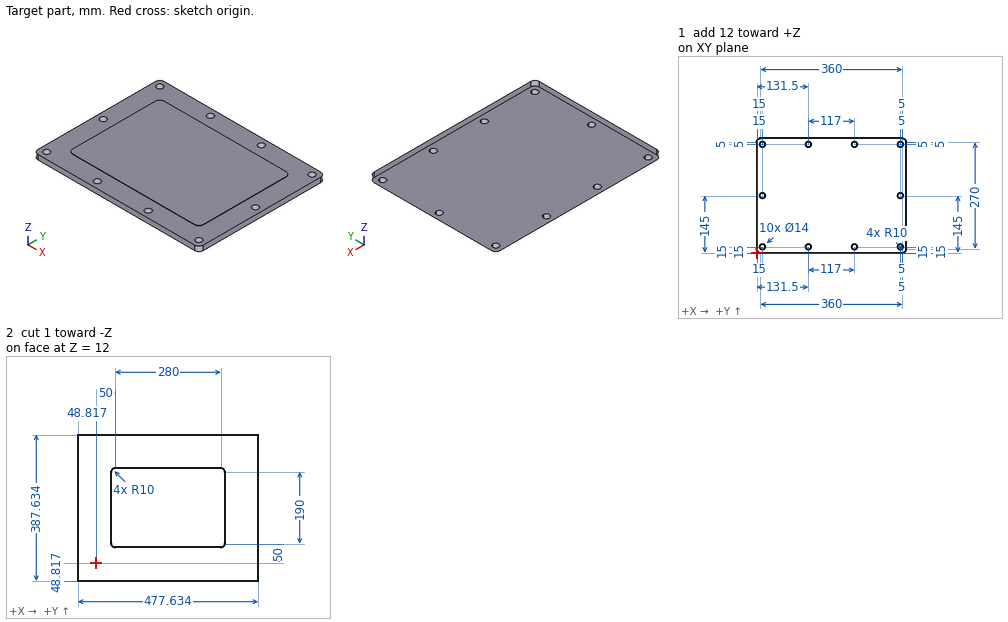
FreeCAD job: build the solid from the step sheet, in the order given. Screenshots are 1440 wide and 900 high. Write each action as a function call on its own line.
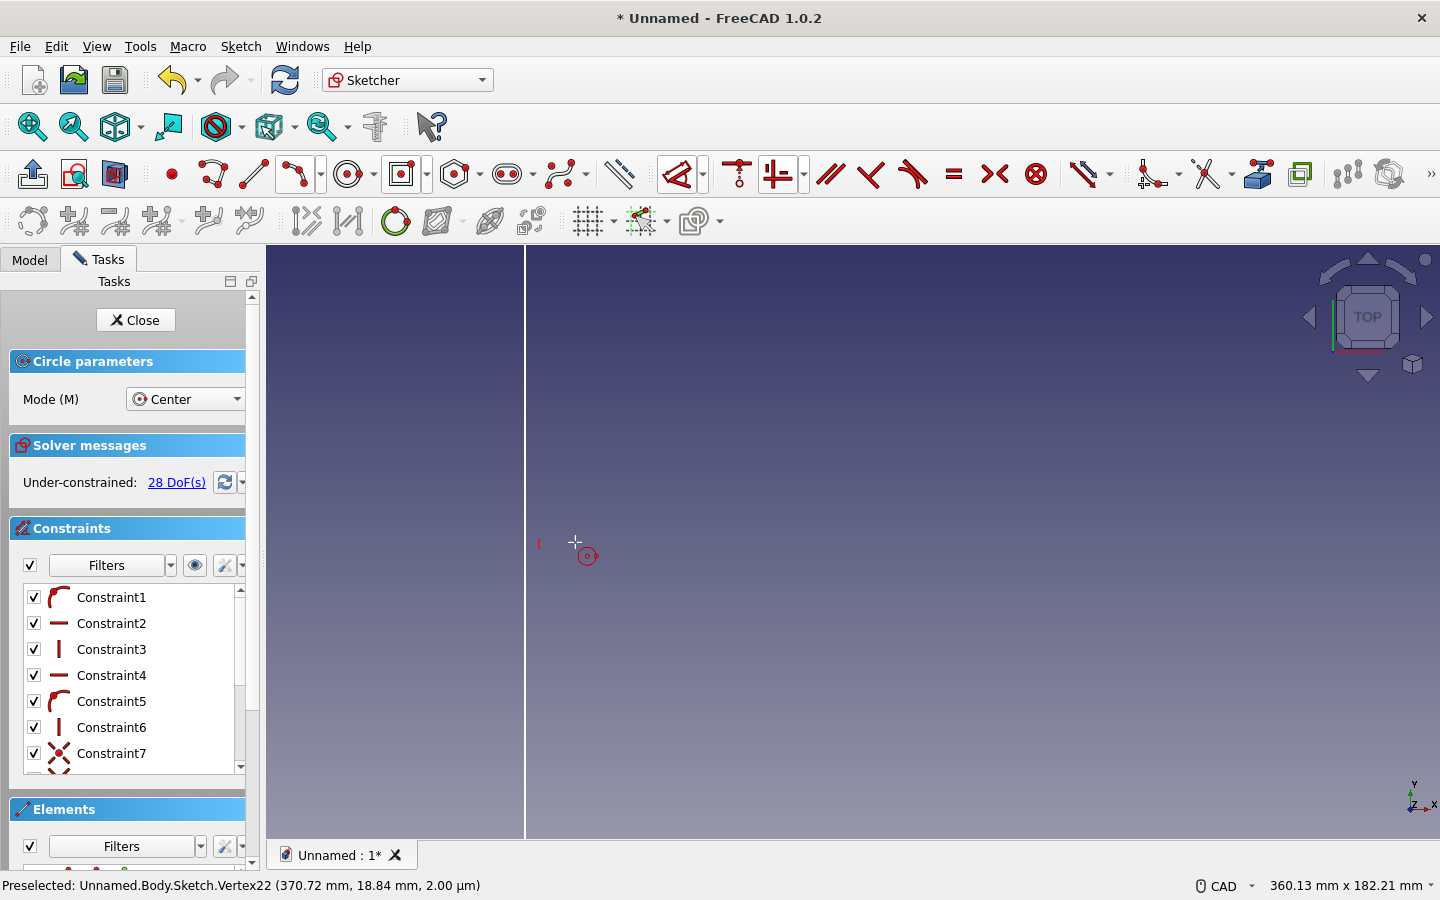
click(574, 542)
click(590, 526)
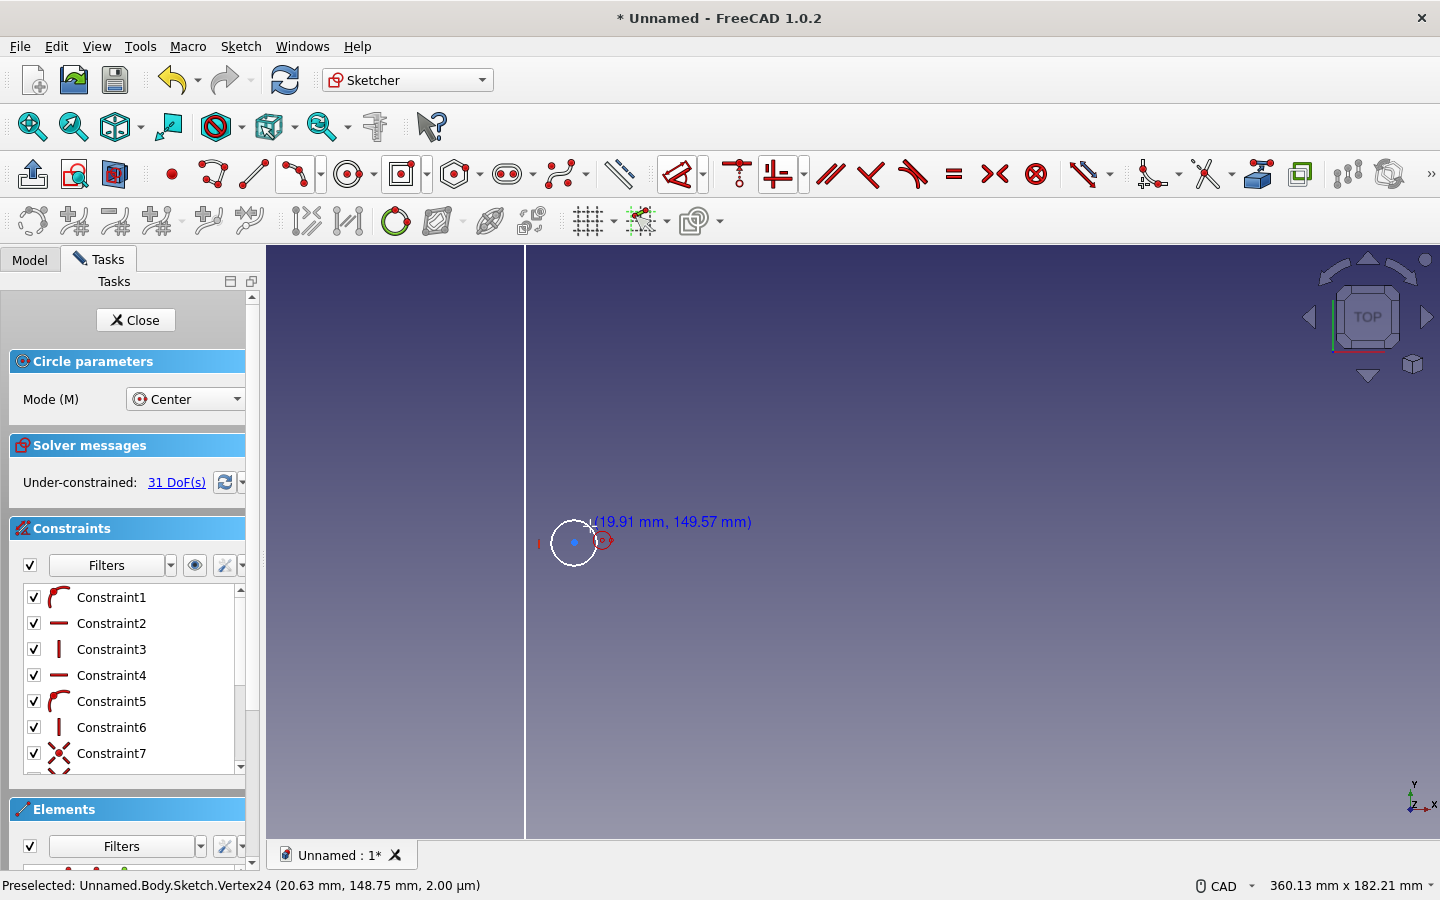
scroll(575, 542, down, 5)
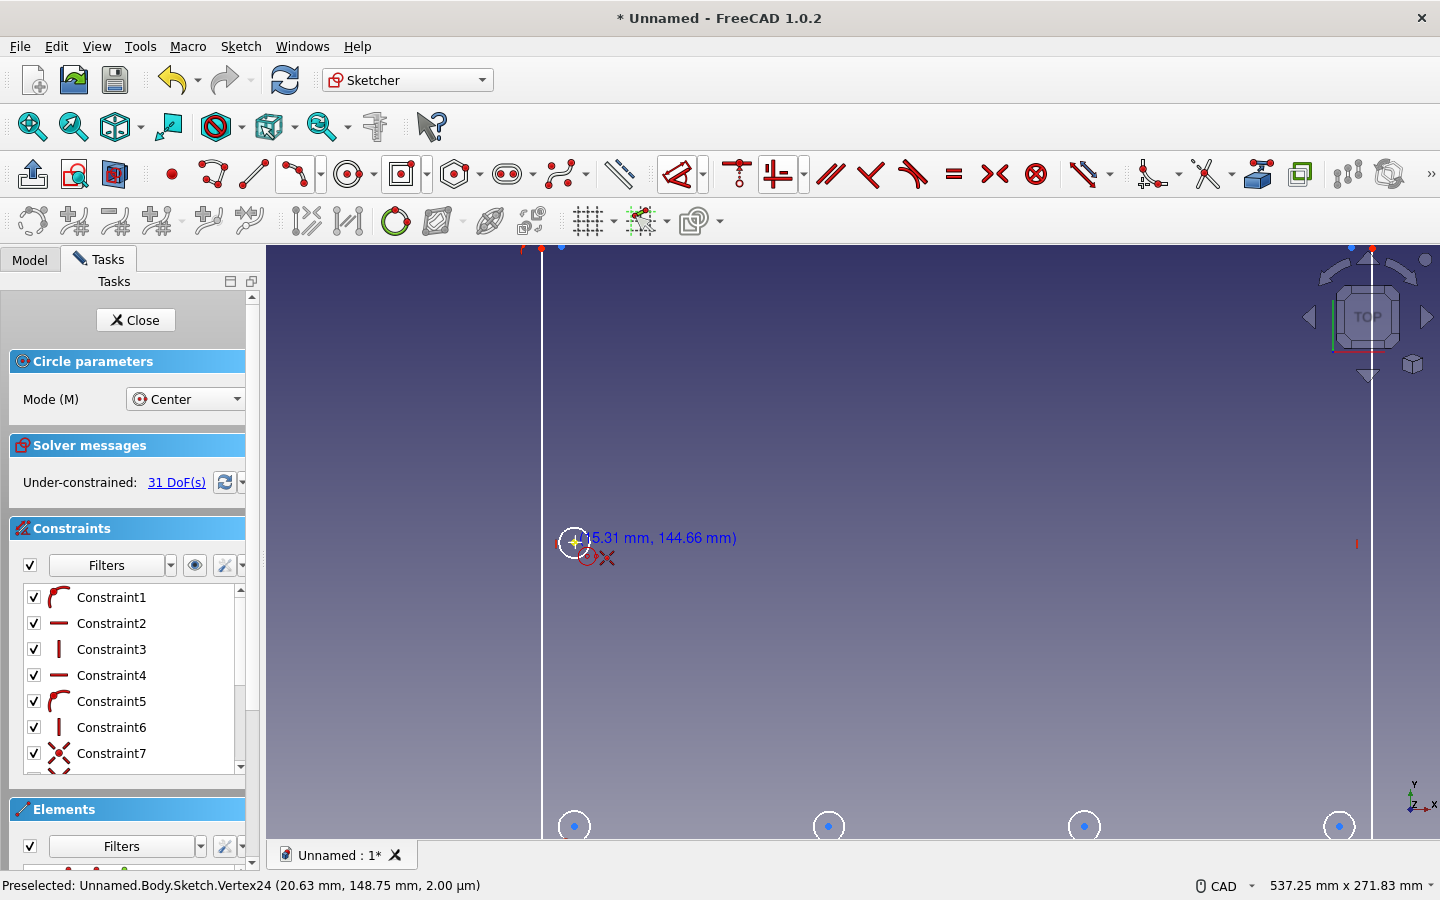
scroll(575, 386, up, 5)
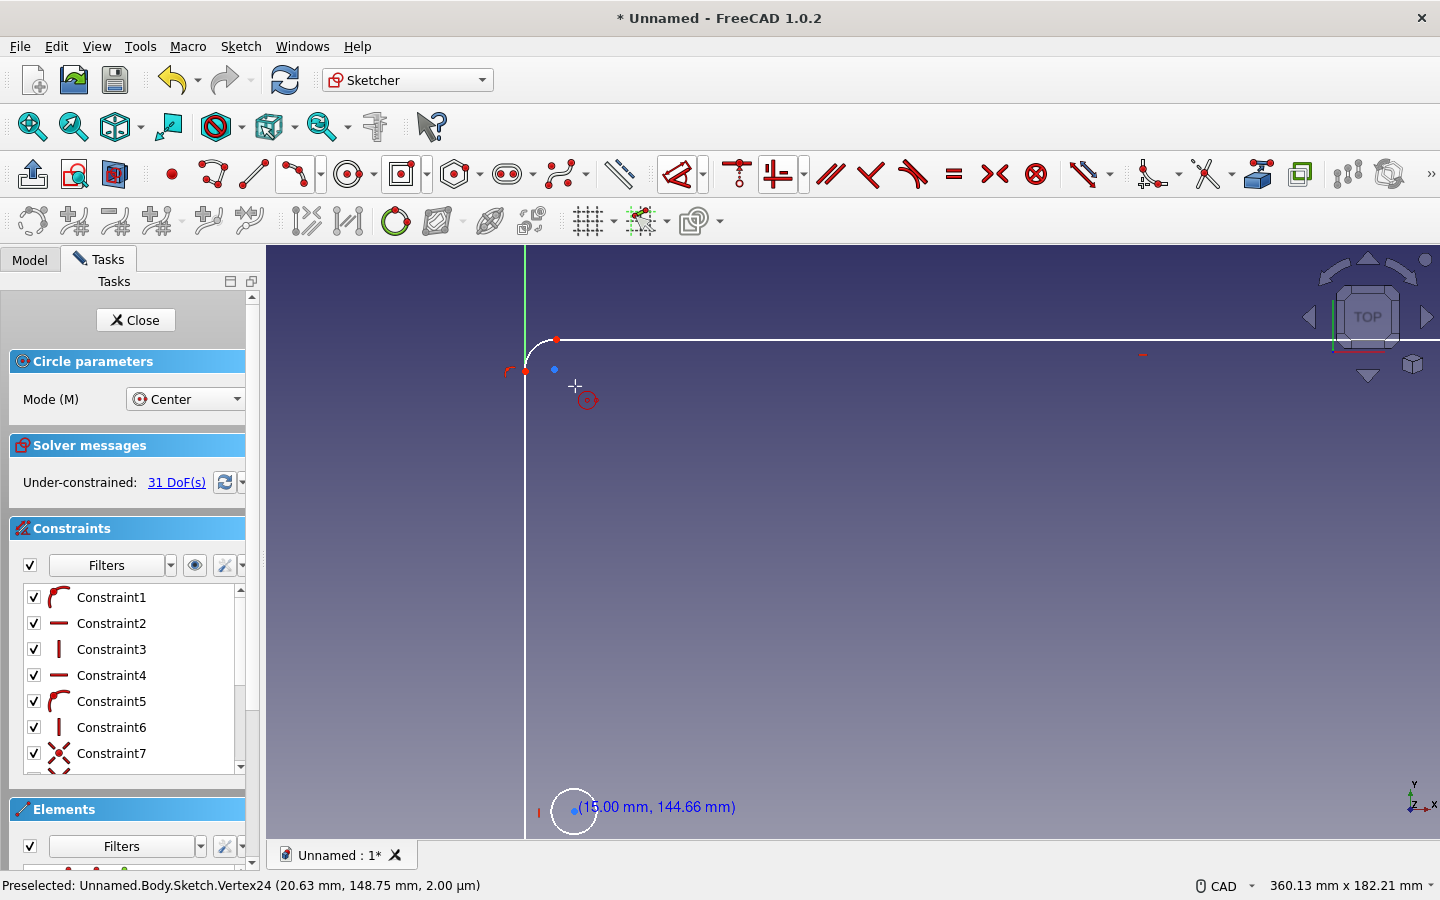
click(574, 387)
click(590, 370)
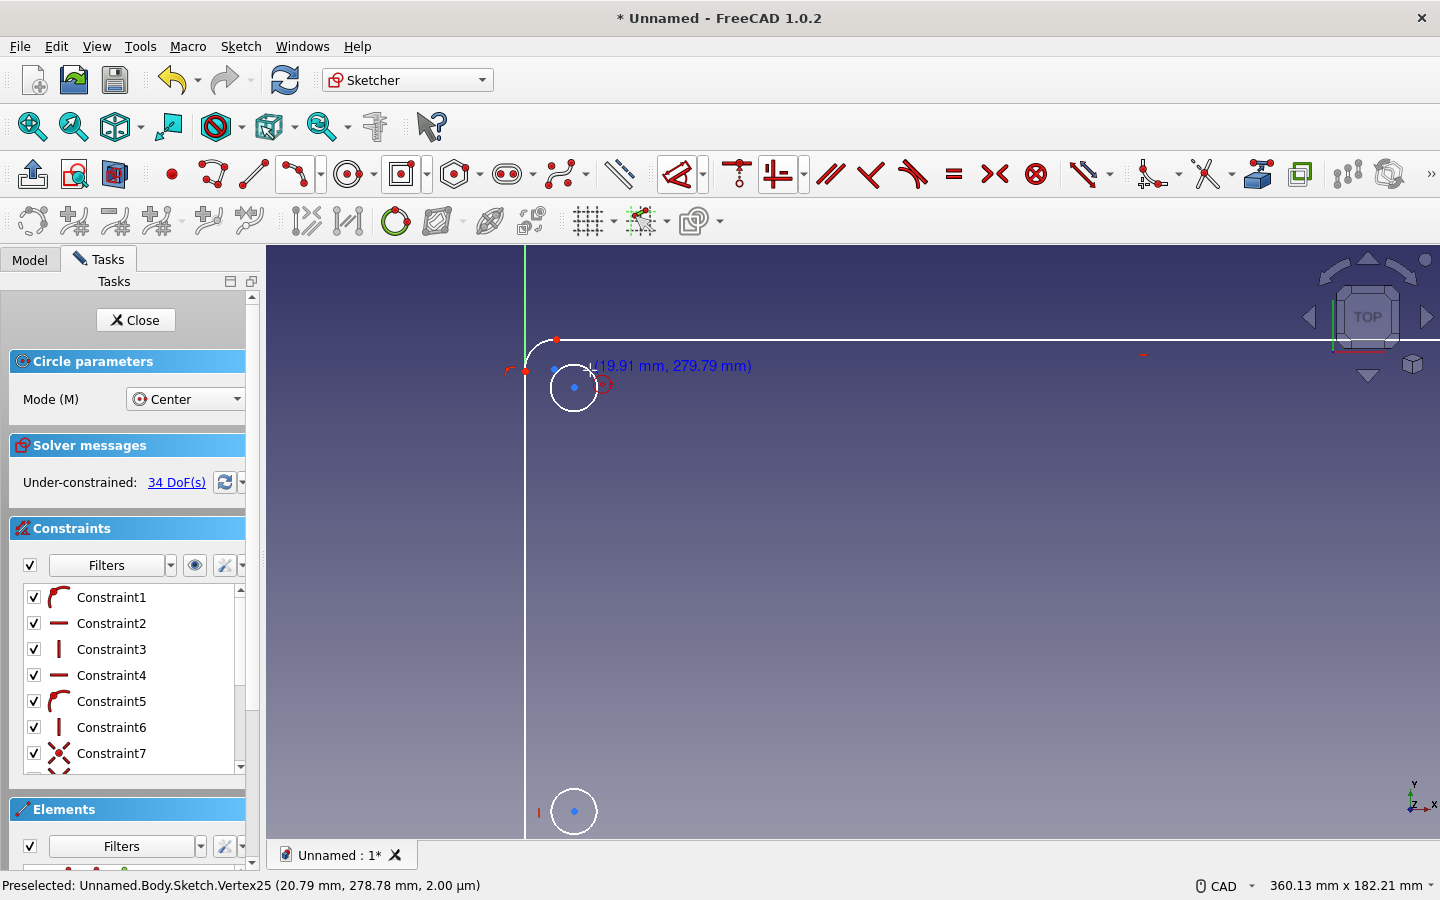
click(954, 387)
click(970, 370)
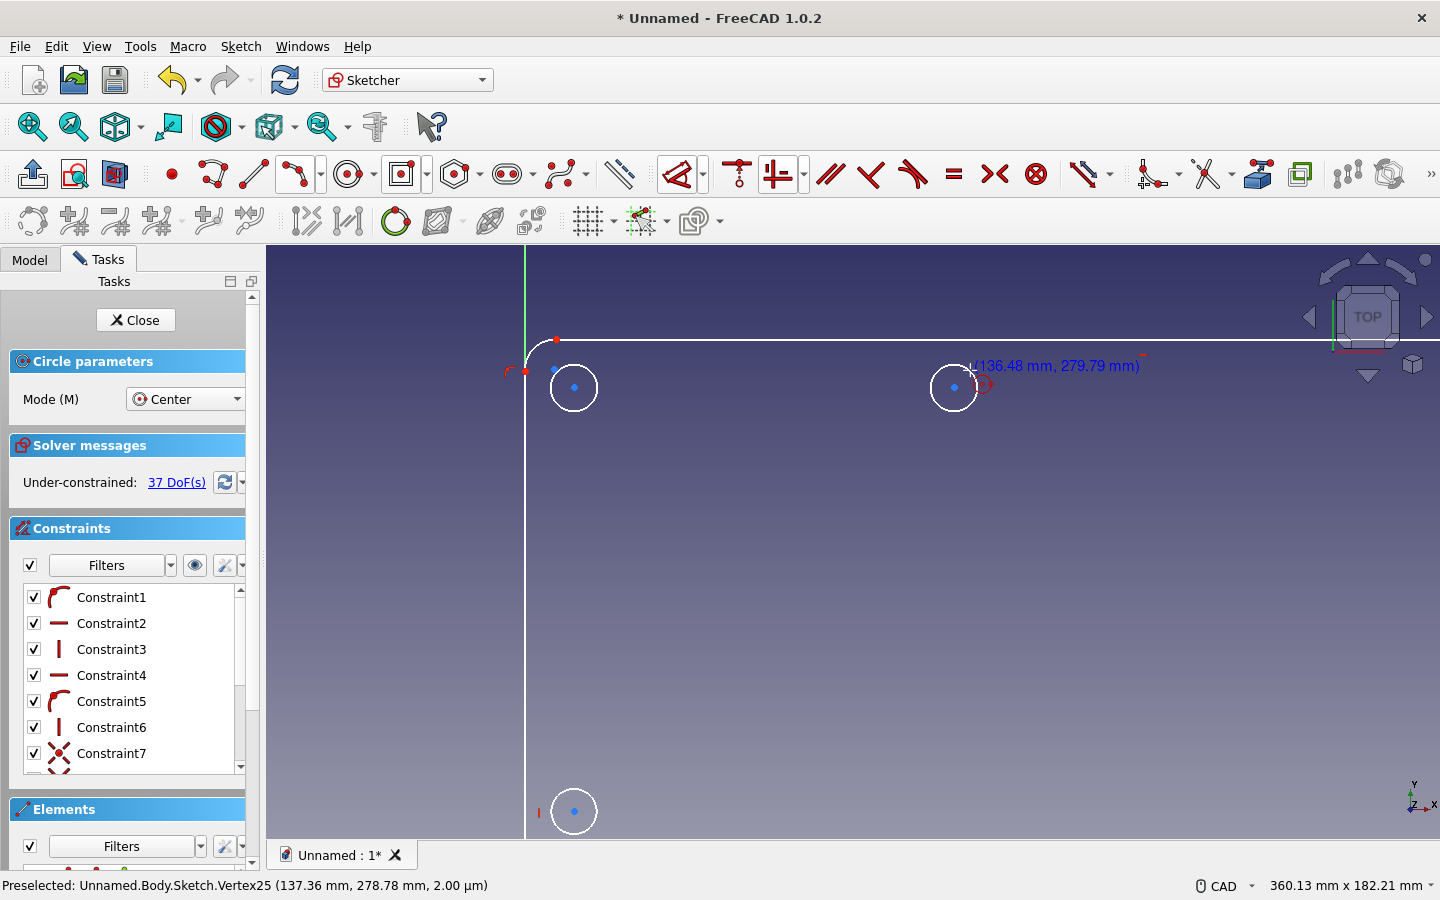
scroll(575, 386, down, 5)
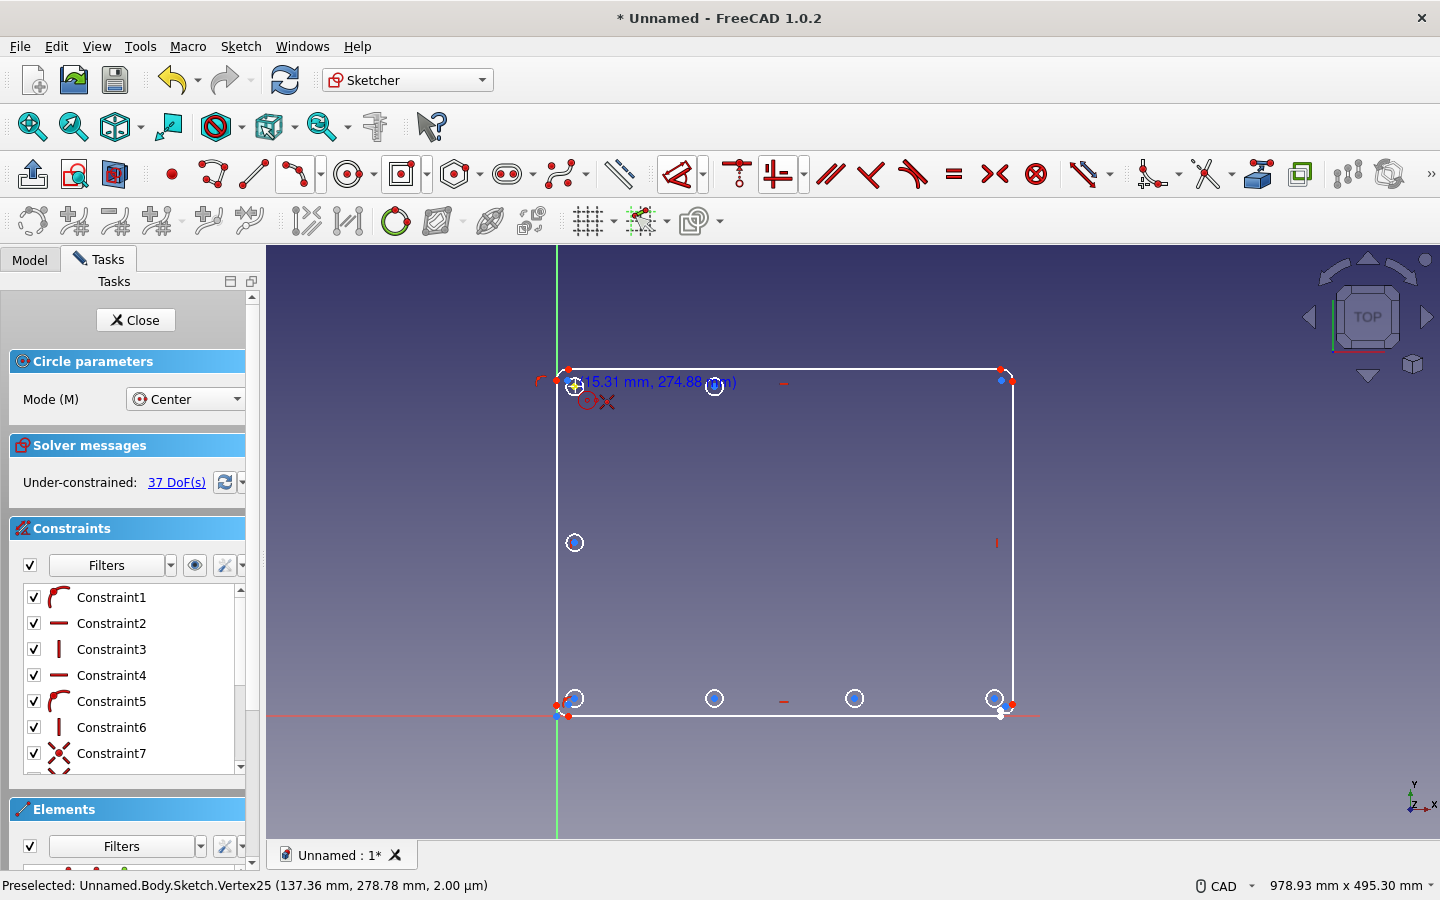
scroll(995, 542, up, 5)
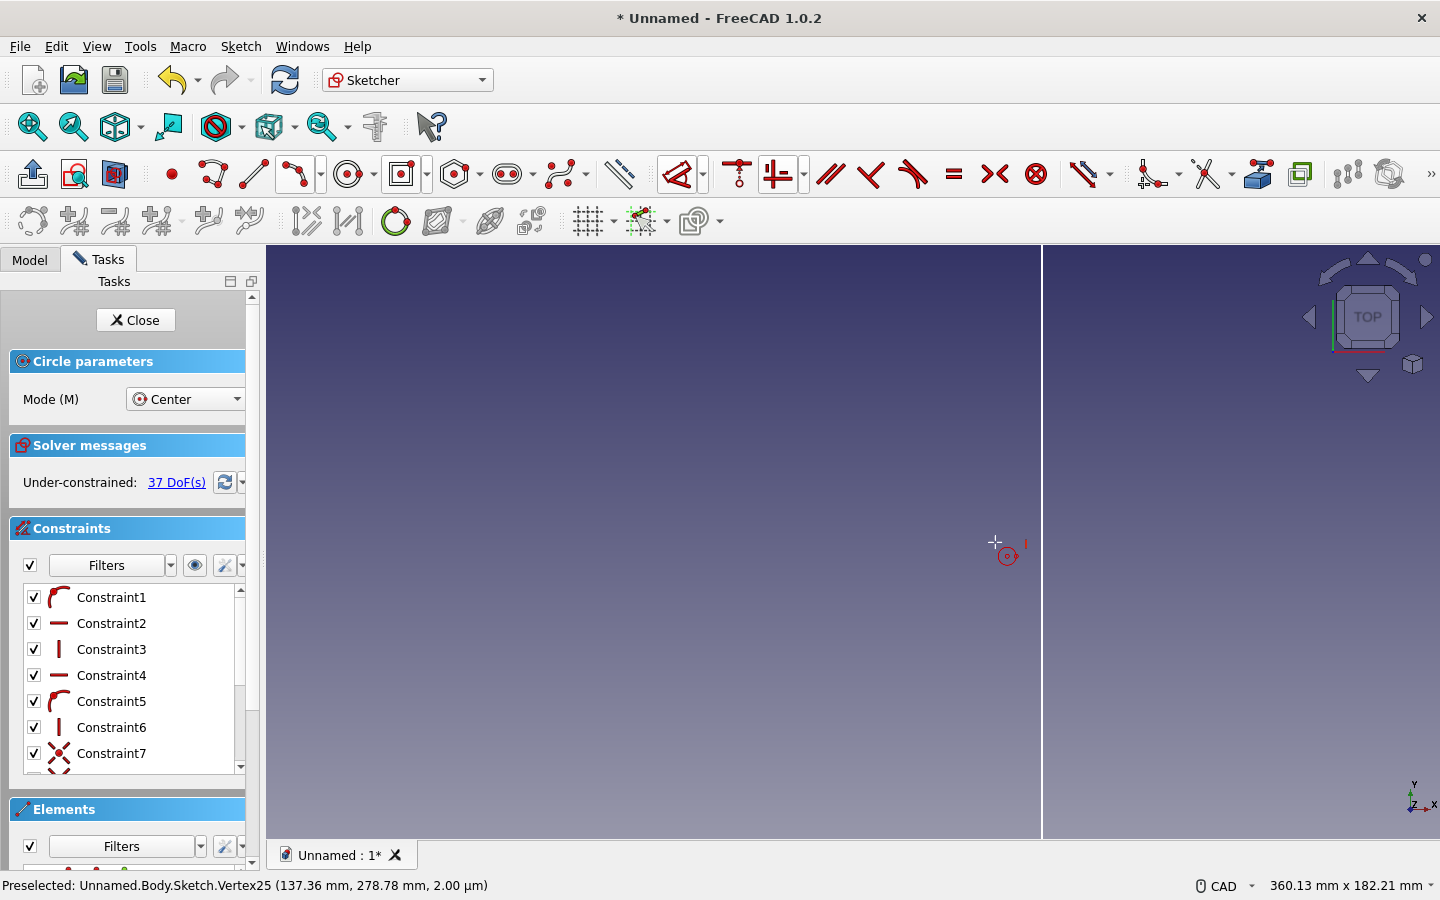
click(993, 542)
click(1009, 526)